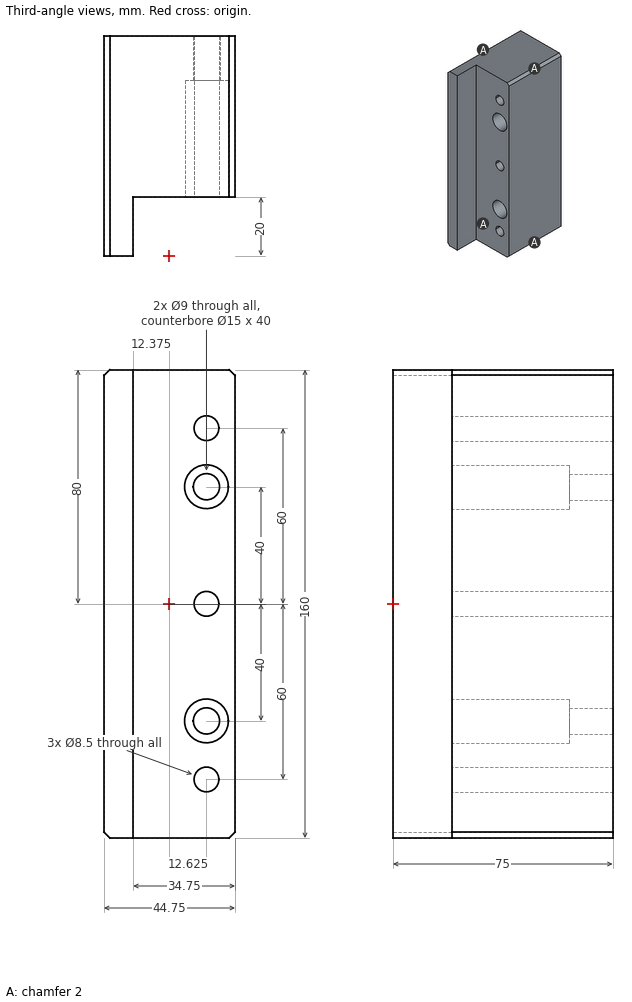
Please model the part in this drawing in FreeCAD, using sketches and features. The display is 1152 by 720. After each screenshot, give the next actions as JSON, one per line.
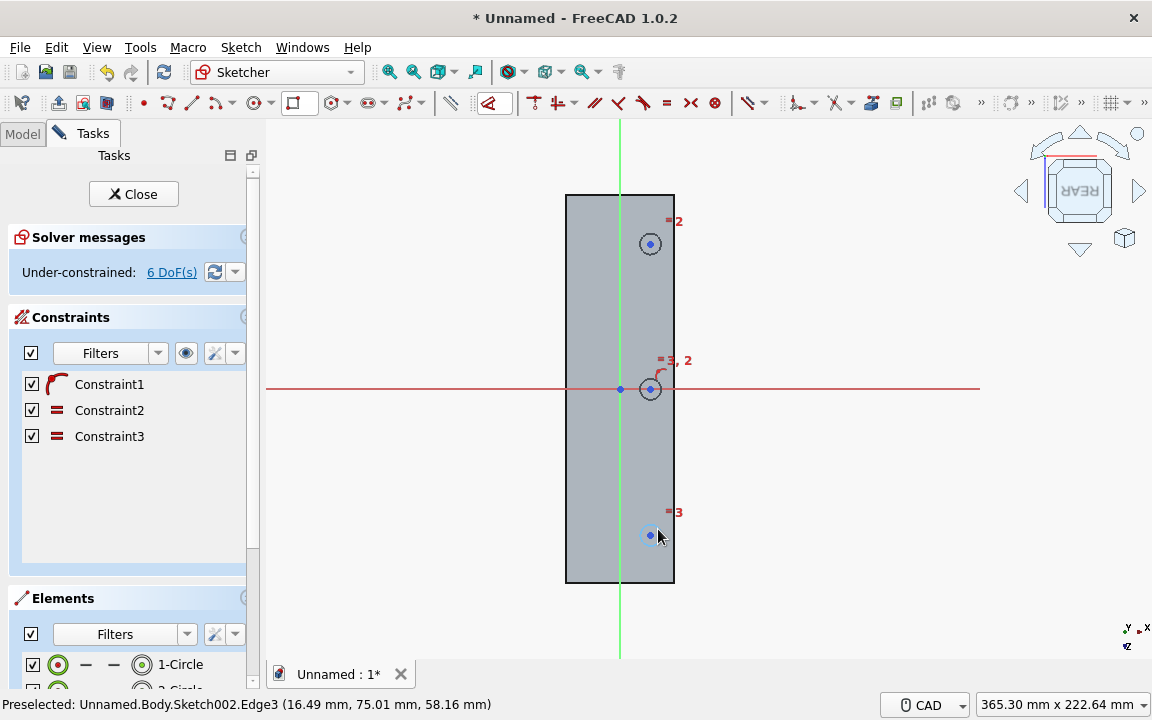
{"action": "left_click", "coordinate": [651, 244]}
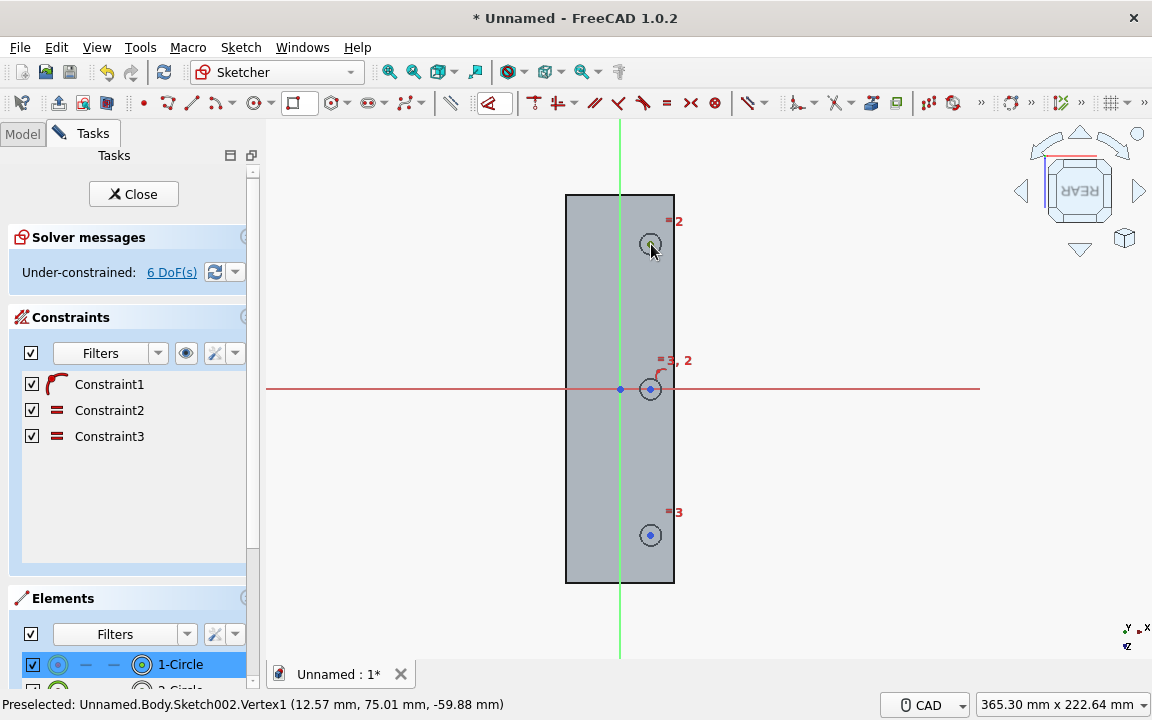
{"action": "left_click", "coordinate": [651, 389]}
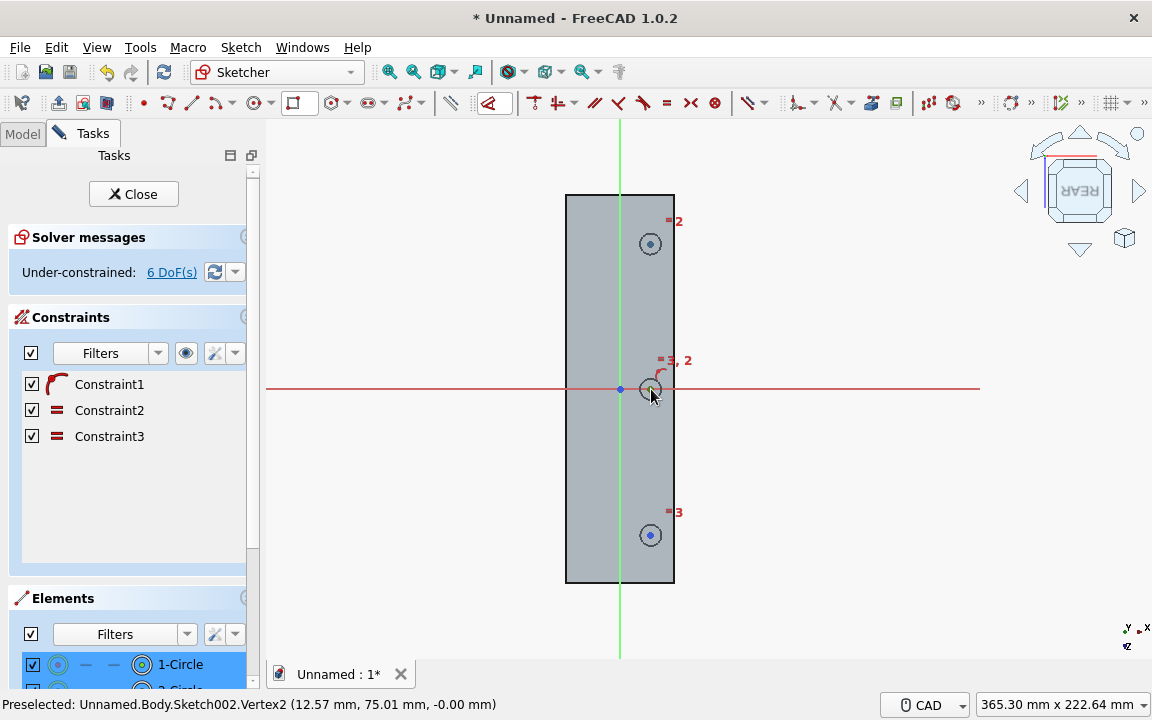
{"action": "key", "text": "v"}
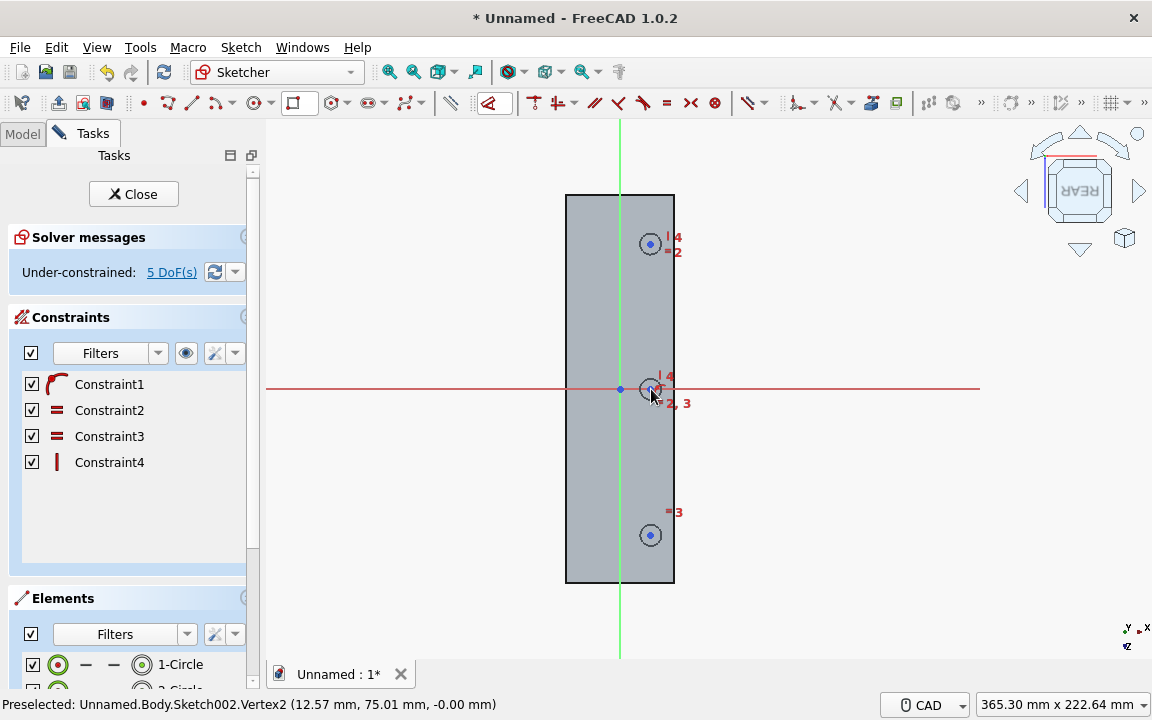
{"action": "left_click", "coordinate": [651, 389]}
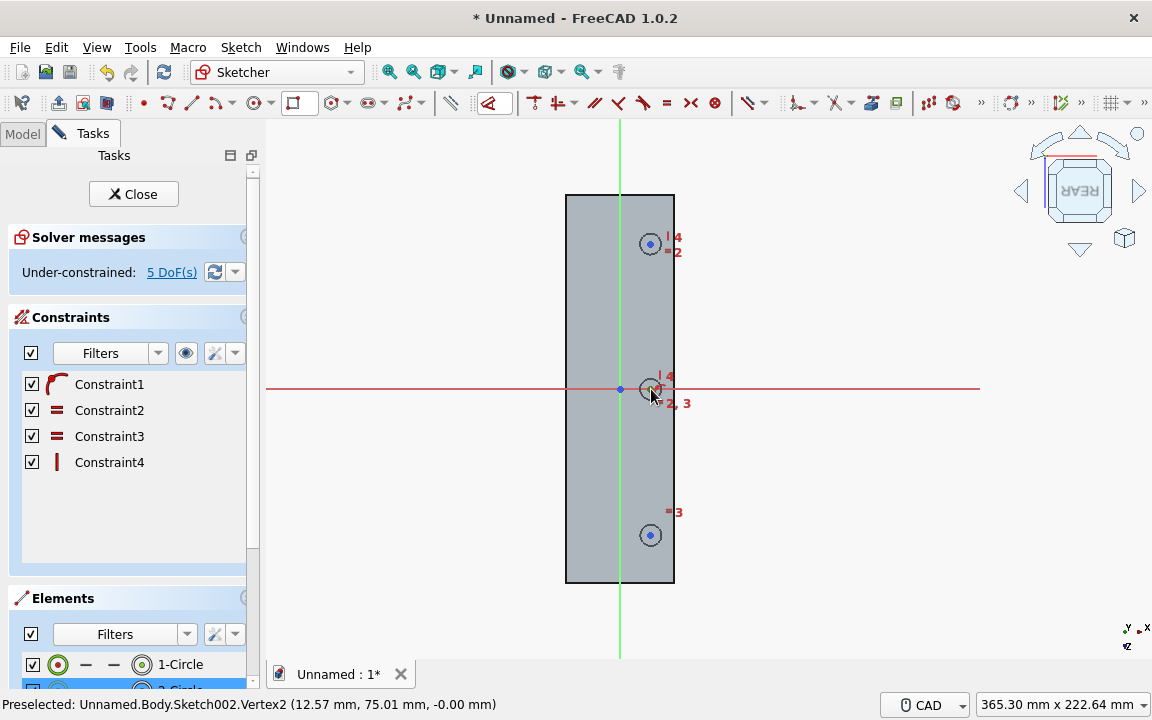
{"action": "left_click", "coordinate": [651, 535]}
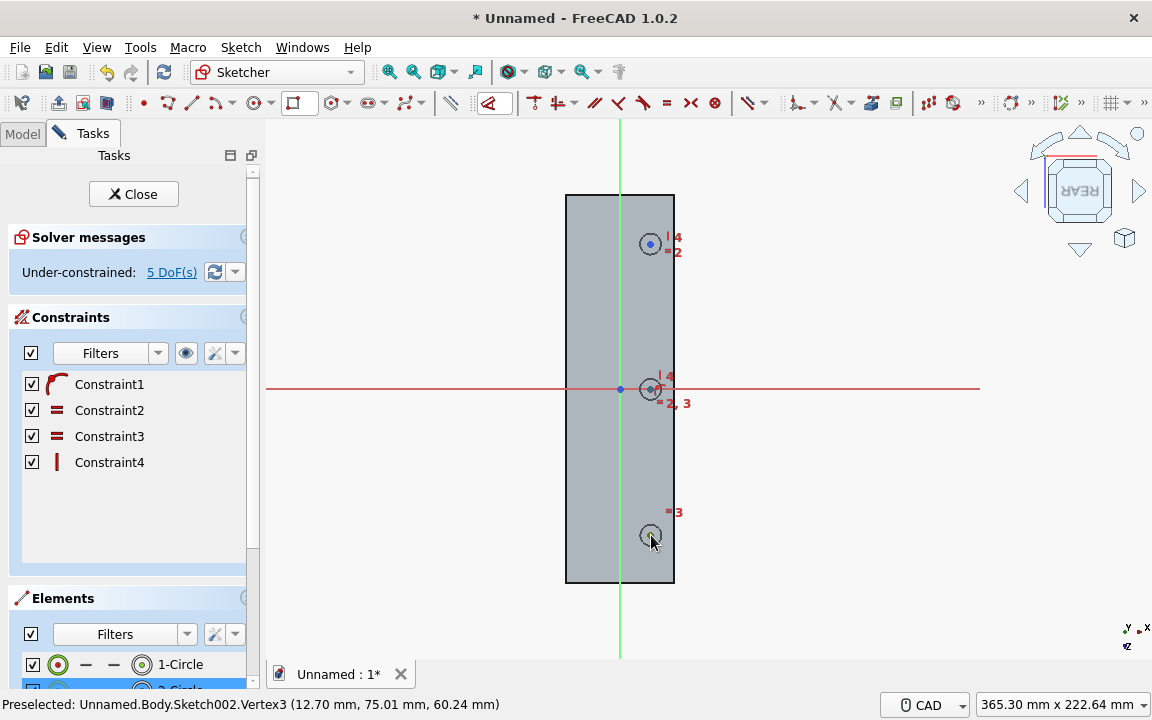
{"action": "key", "text": "v"}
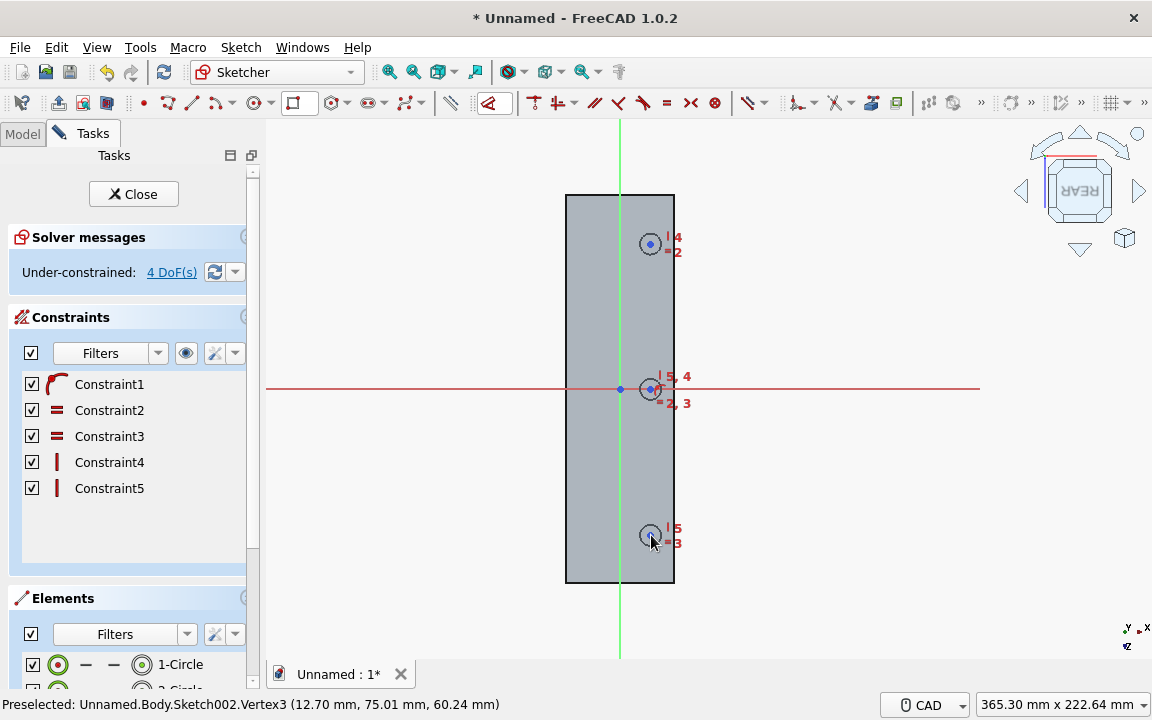
{"action": "key", "text": "d"}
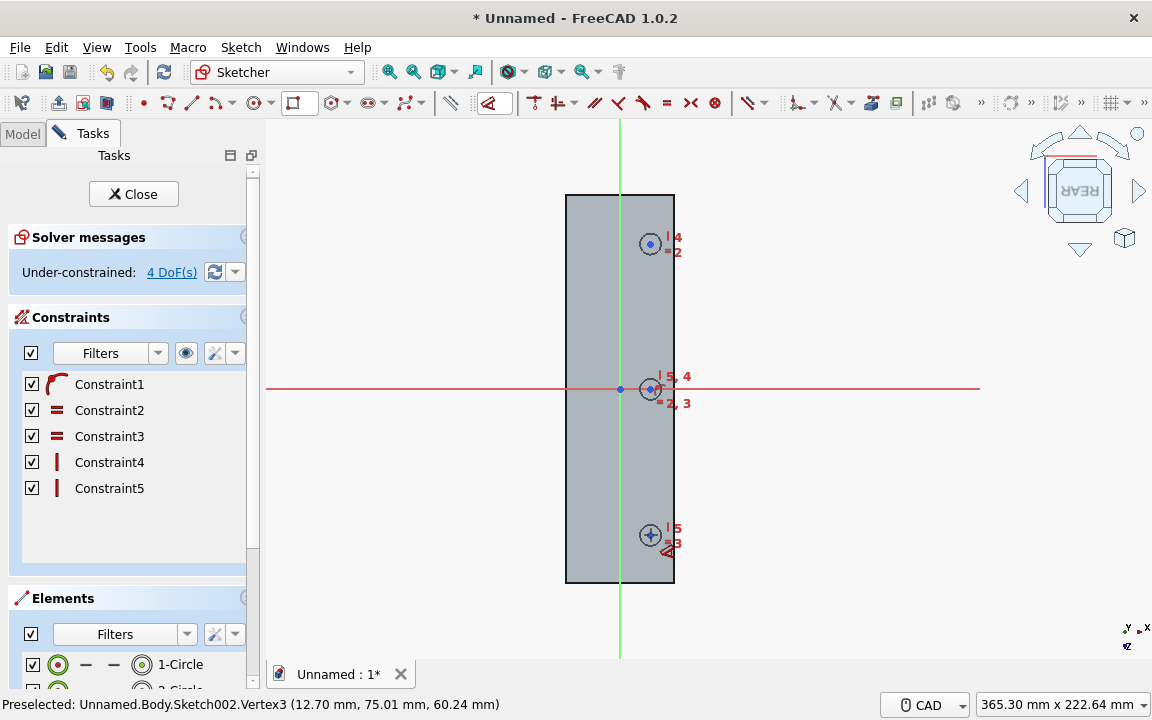
{"action": "scroll", "coordinate": [658, 237], "scroll_direction": "up", "scroll_amount": 4}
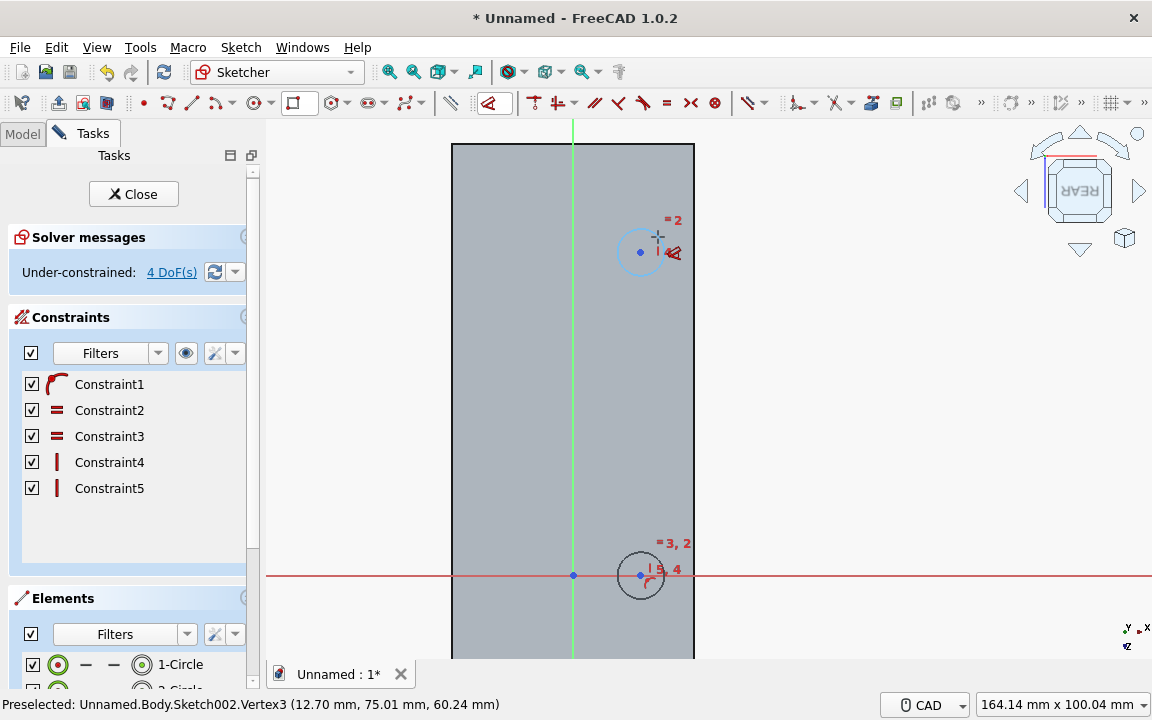
{"action": "left_click", "coordinate": [657, 236]}
{"action": "left_click", "coordinate": [679, 213]}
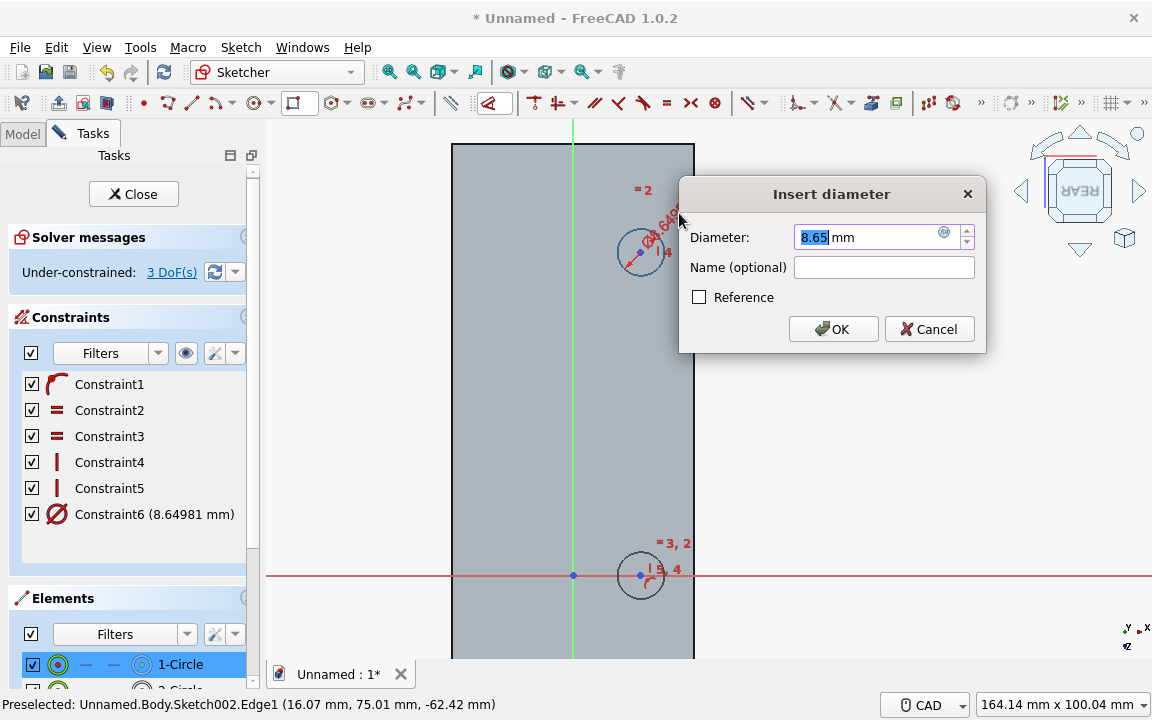
{"action": "type", "text": "8.5"}
{"action": "key", "text": "Return"}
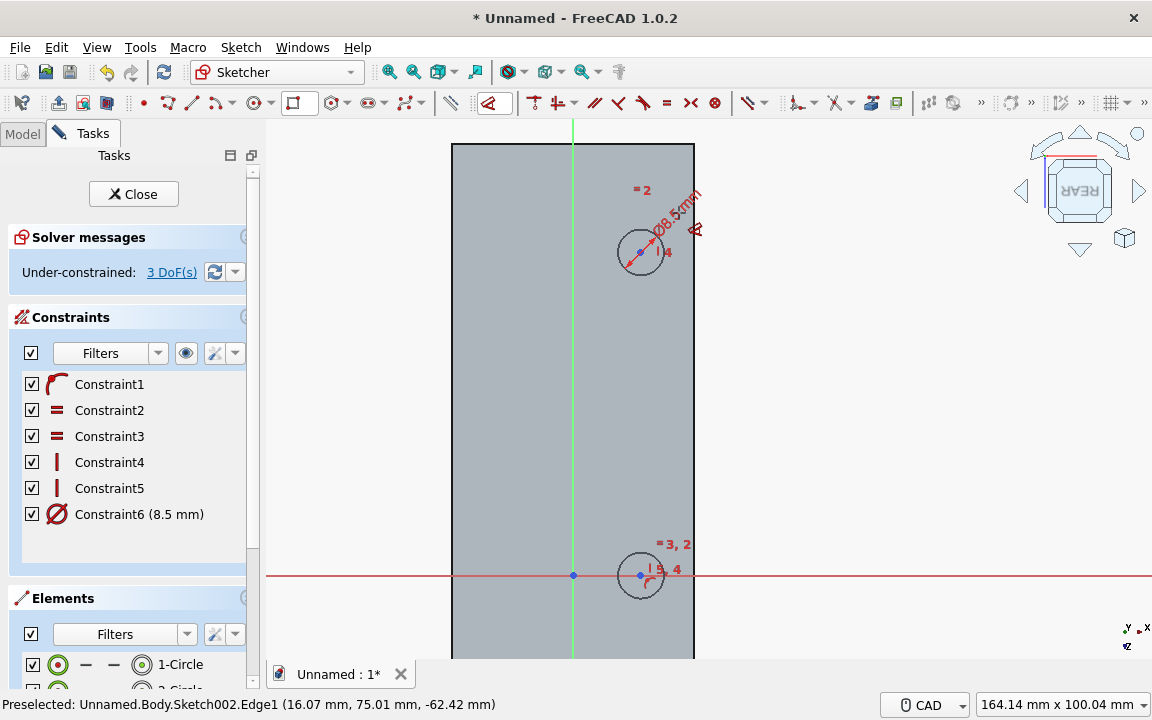
{"action": "left_click", "coordinate": [641, 252]}
{"action": "left_click", "coordinate": [539, 414]}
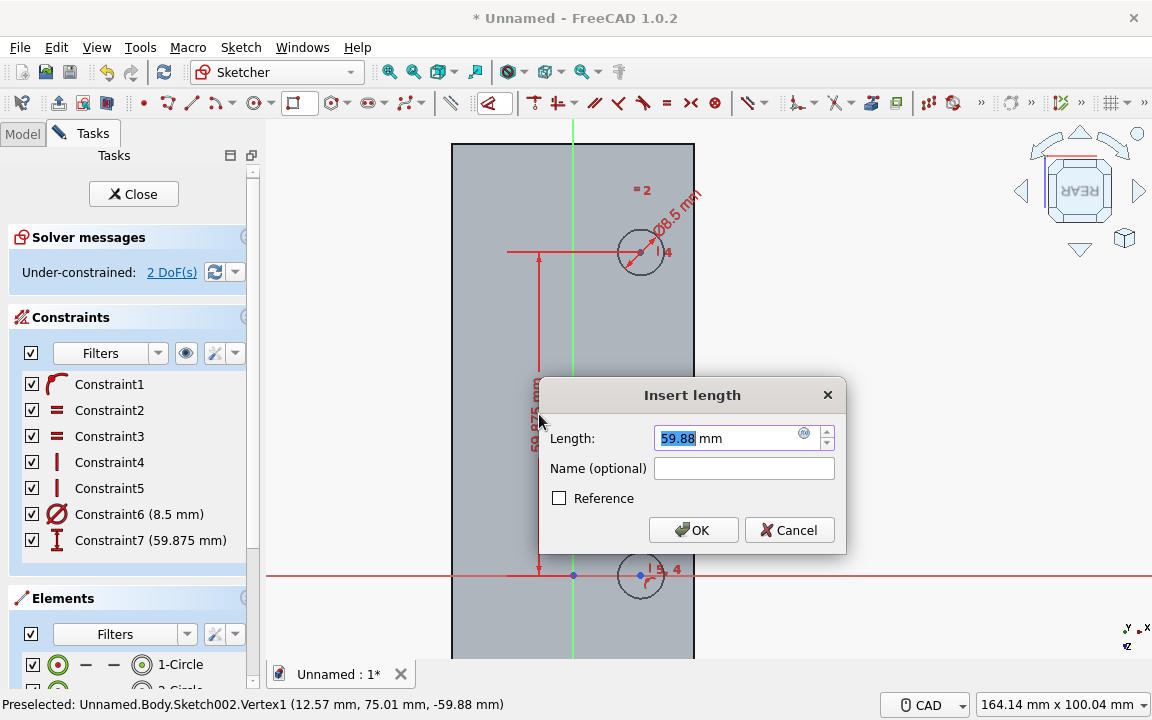
{"action": "type", "text": "60"}
{"action": "key", "text": "Return"}